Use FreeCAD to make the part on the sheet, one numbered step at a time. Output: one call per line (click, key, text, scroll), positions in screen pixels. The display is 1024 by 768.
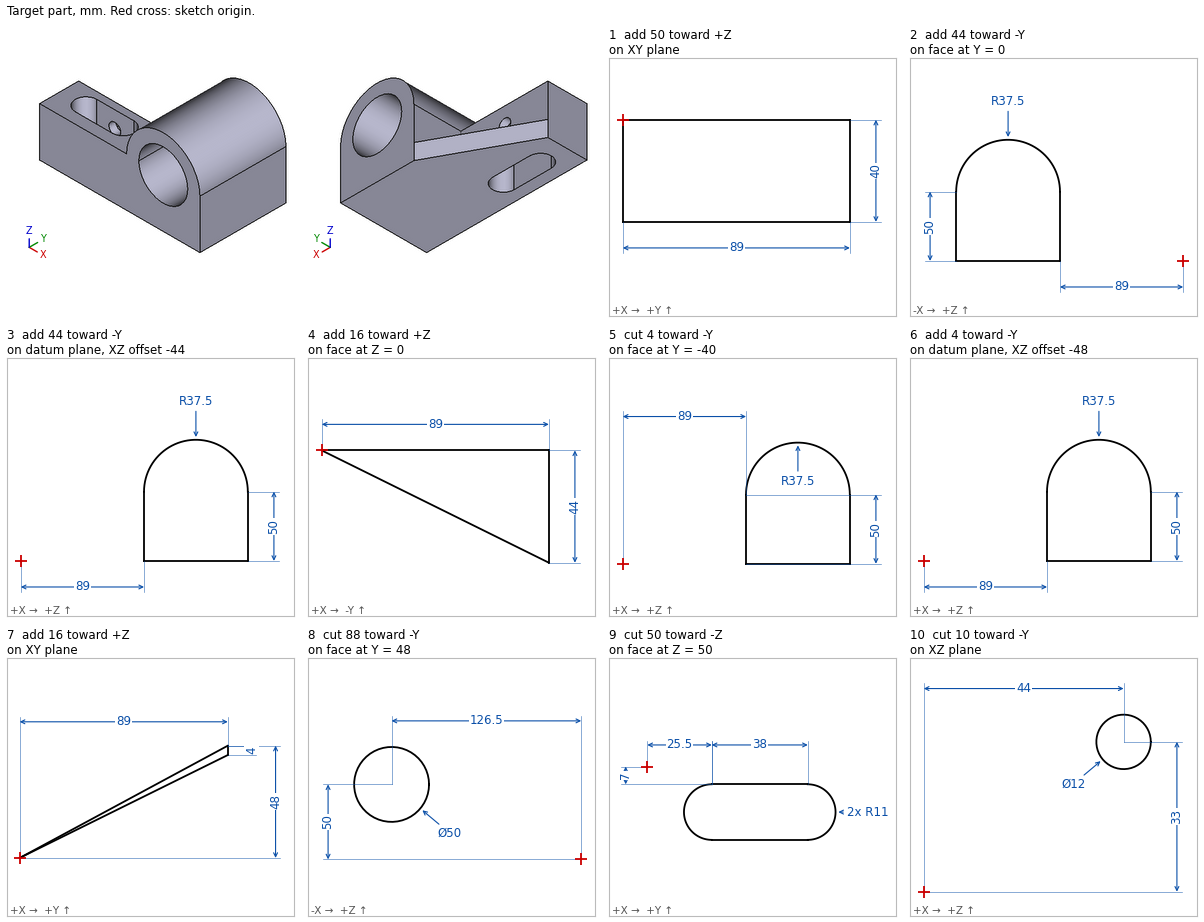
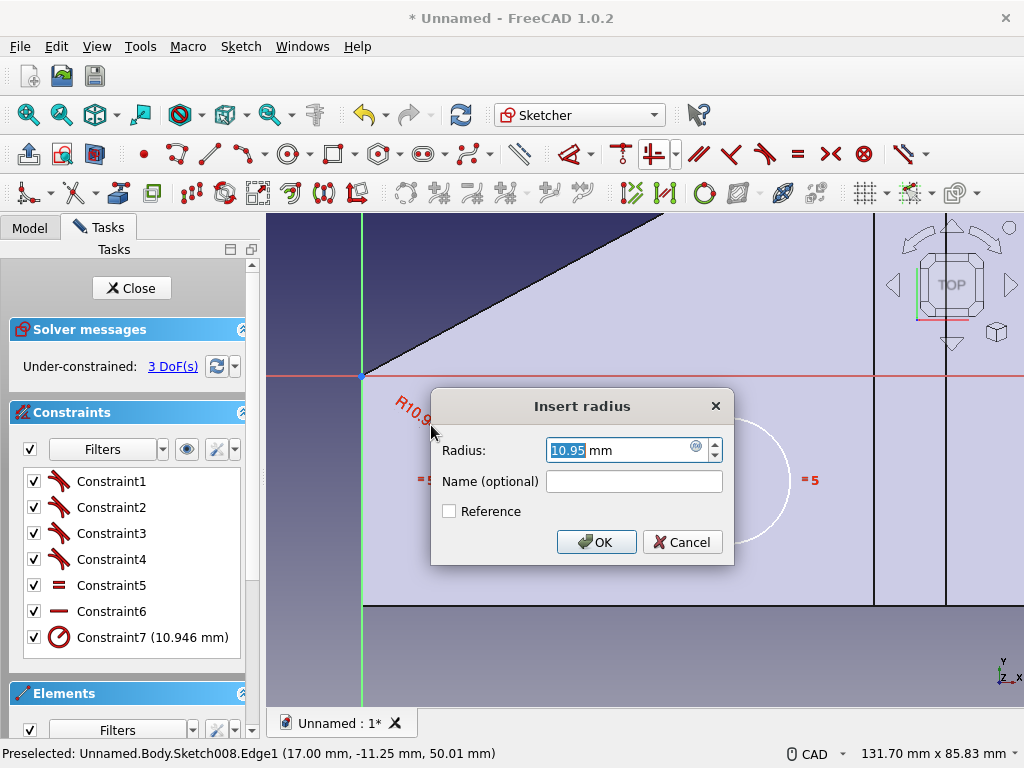
text(11)
key(Return)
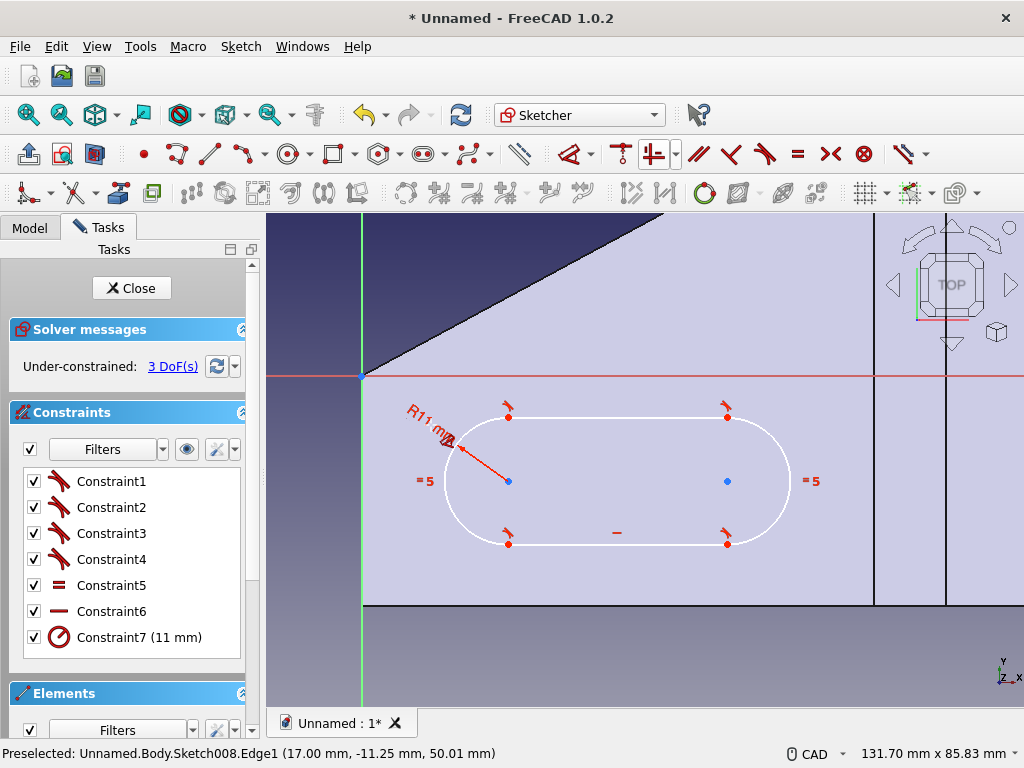
click(574, 418)
click(617, 452)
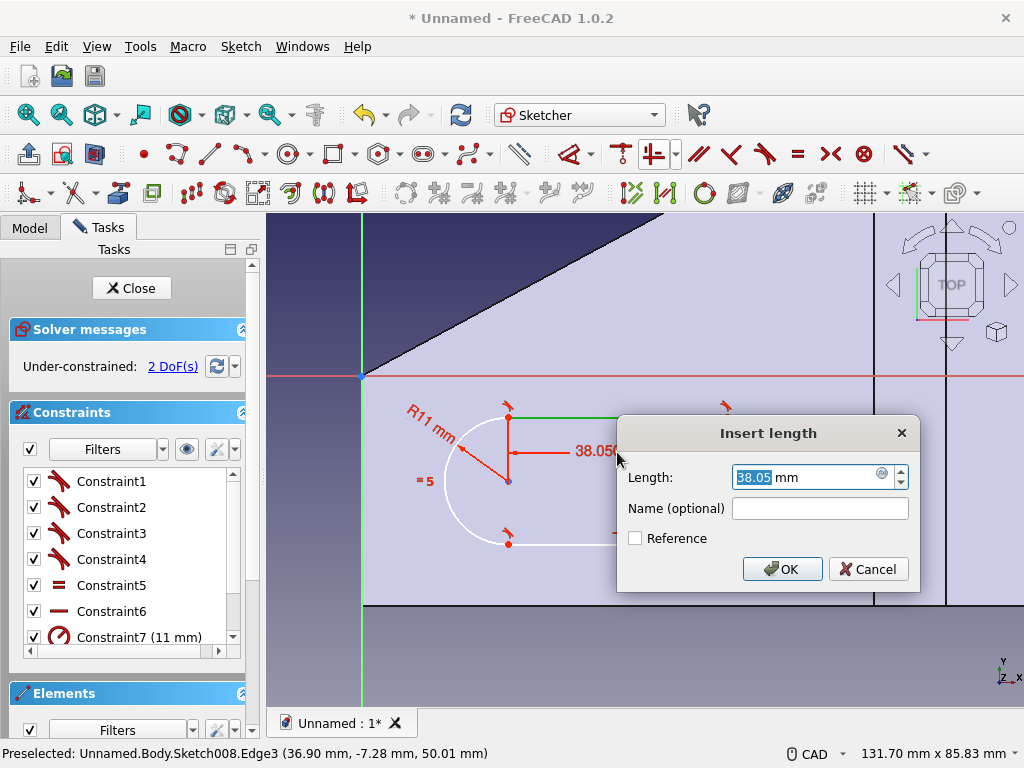
text(38)
key(Return)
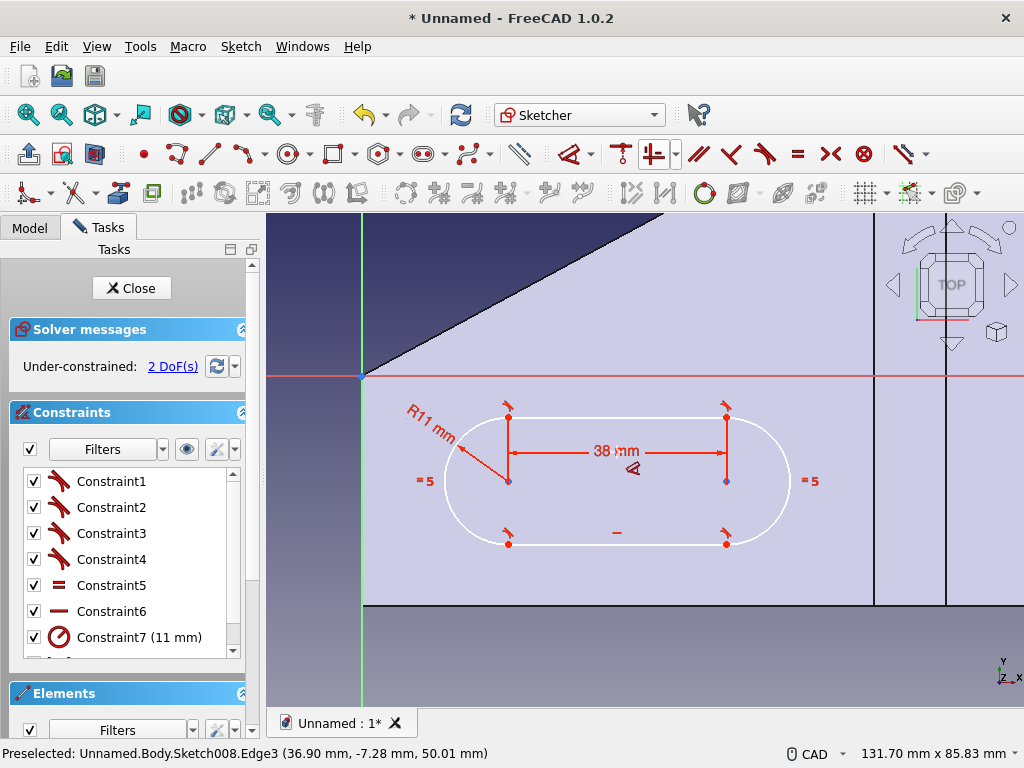
click(508, 418)
click(328, 397)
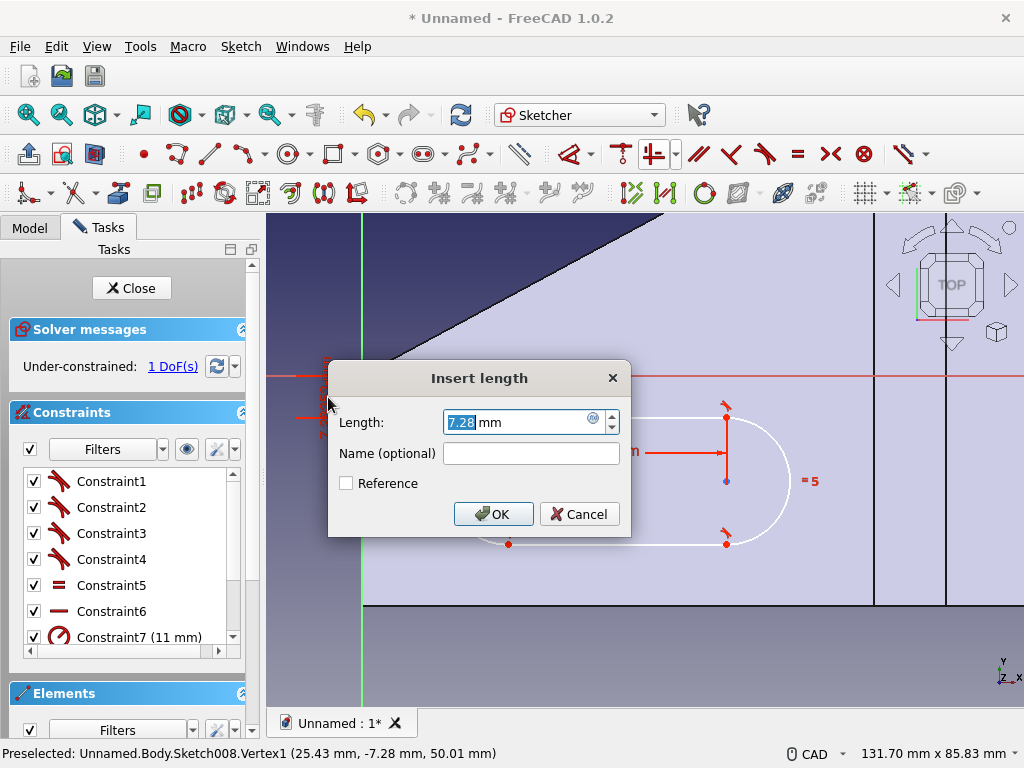
text(7)
key(Return)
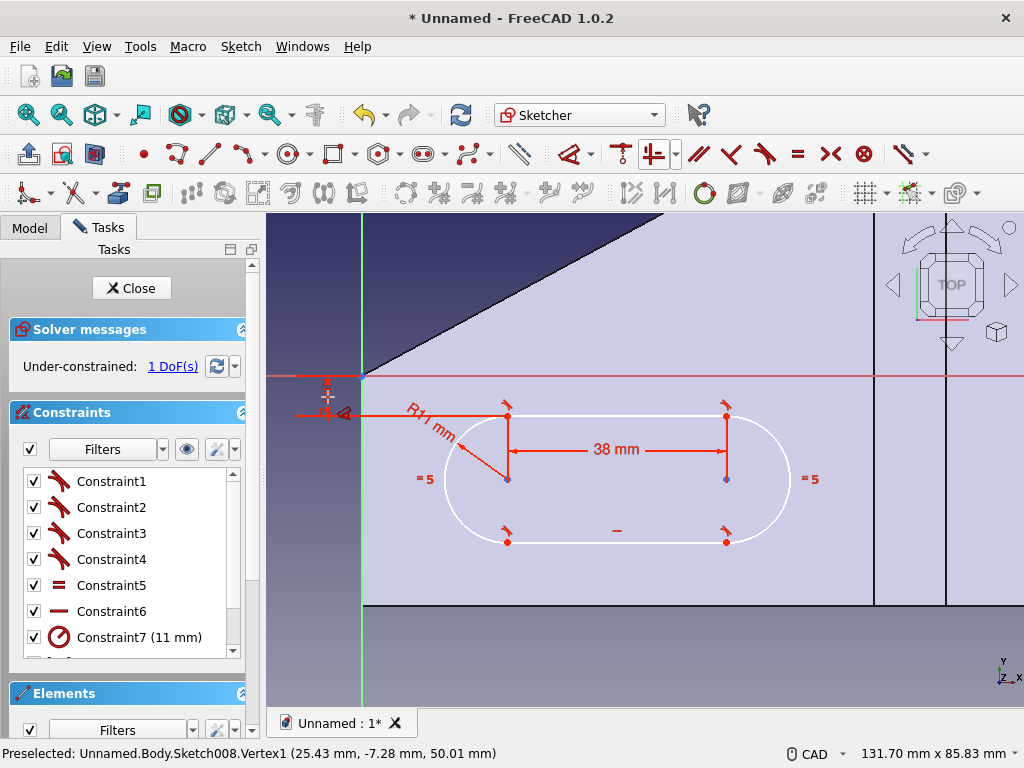
click(508, 416)
click(435, 342)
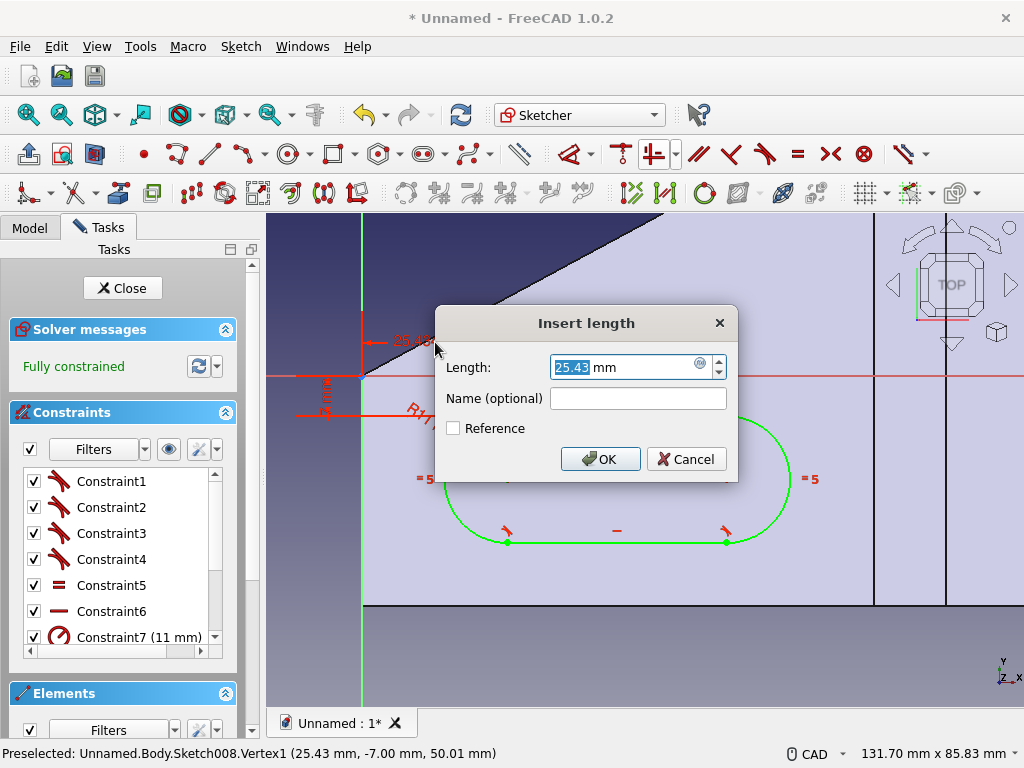
text(25.5)
key(Return)
key(Escape)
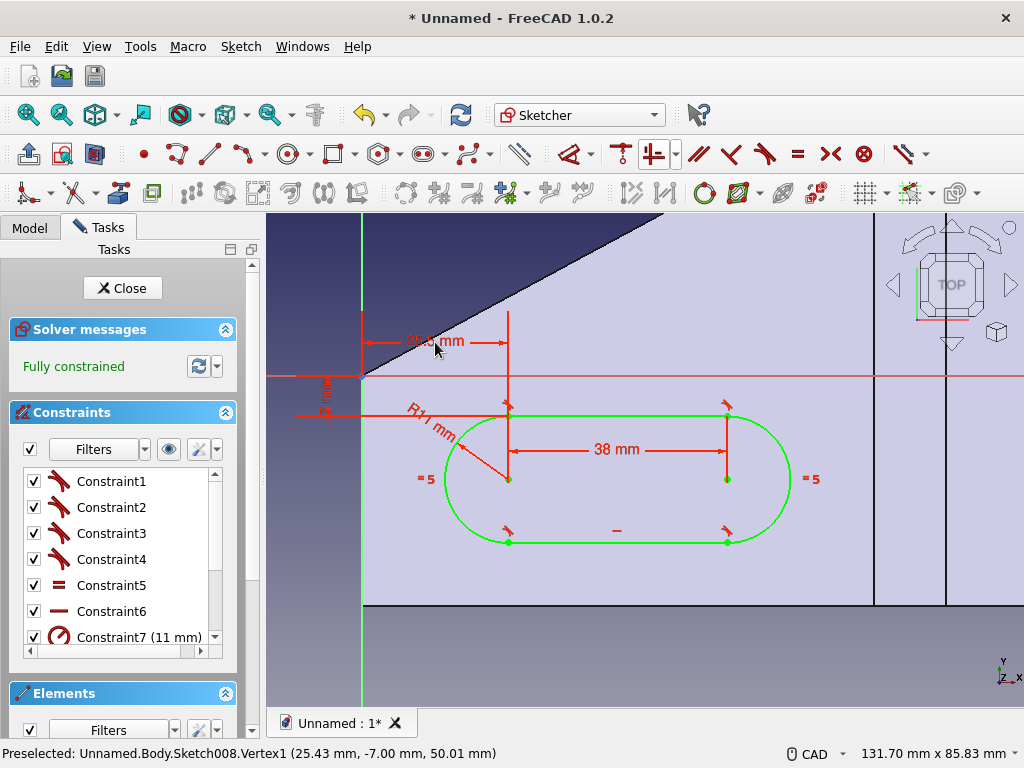
click(123, 288)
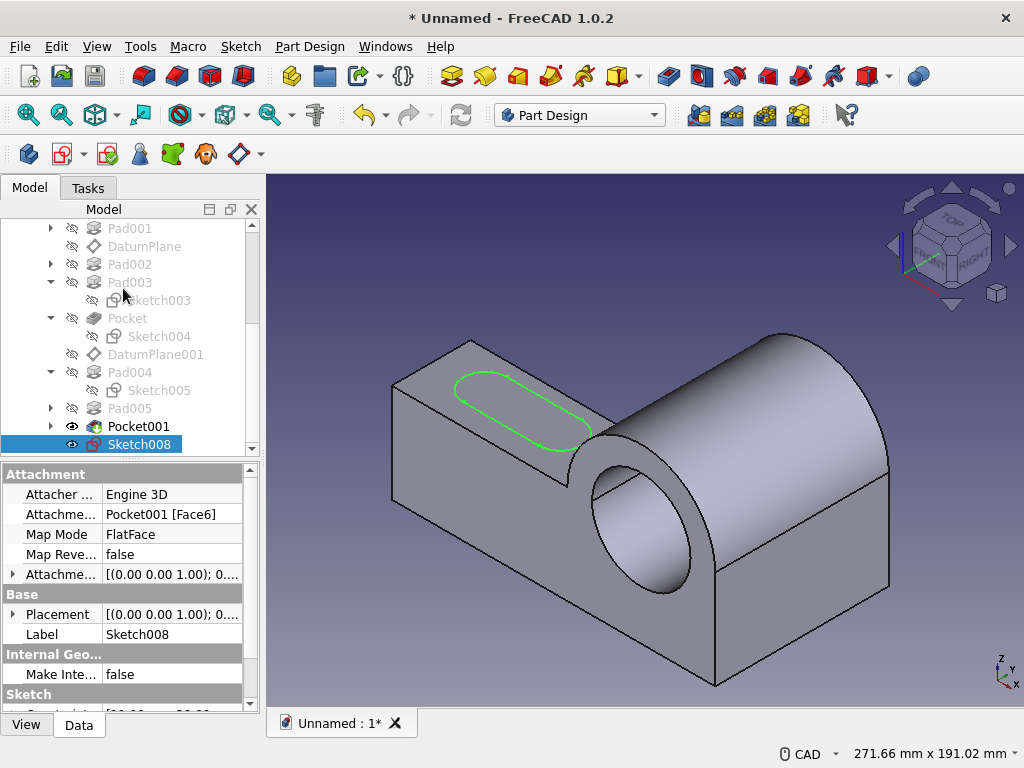
click(669, 76)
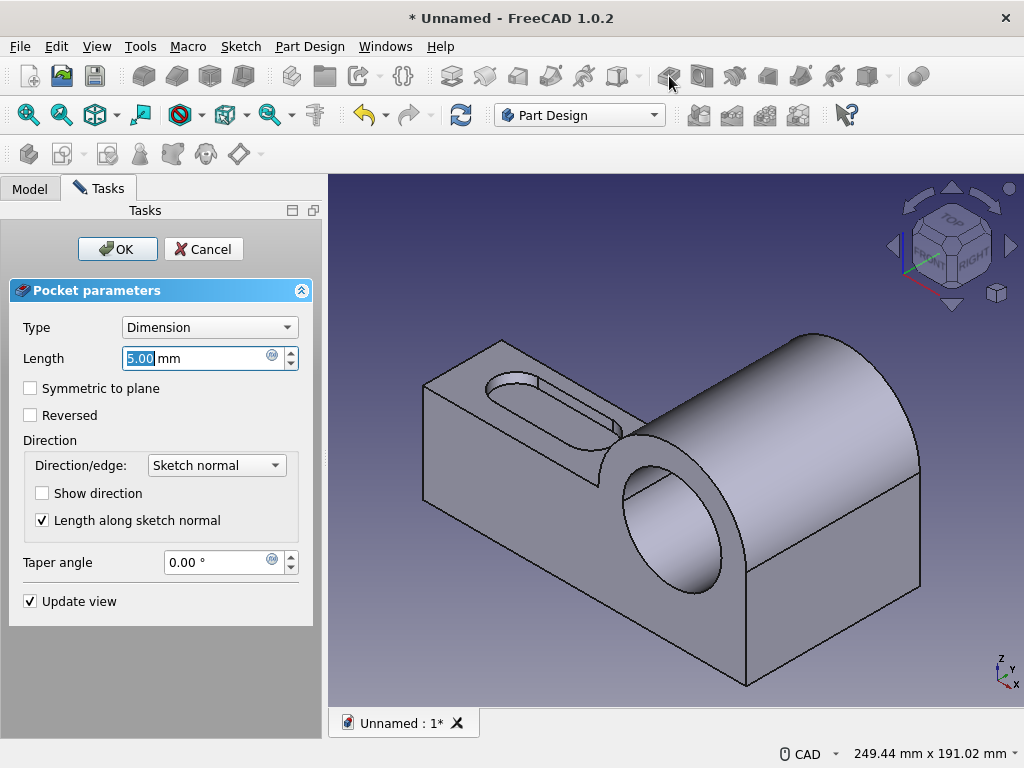
text(50)
key(Tab)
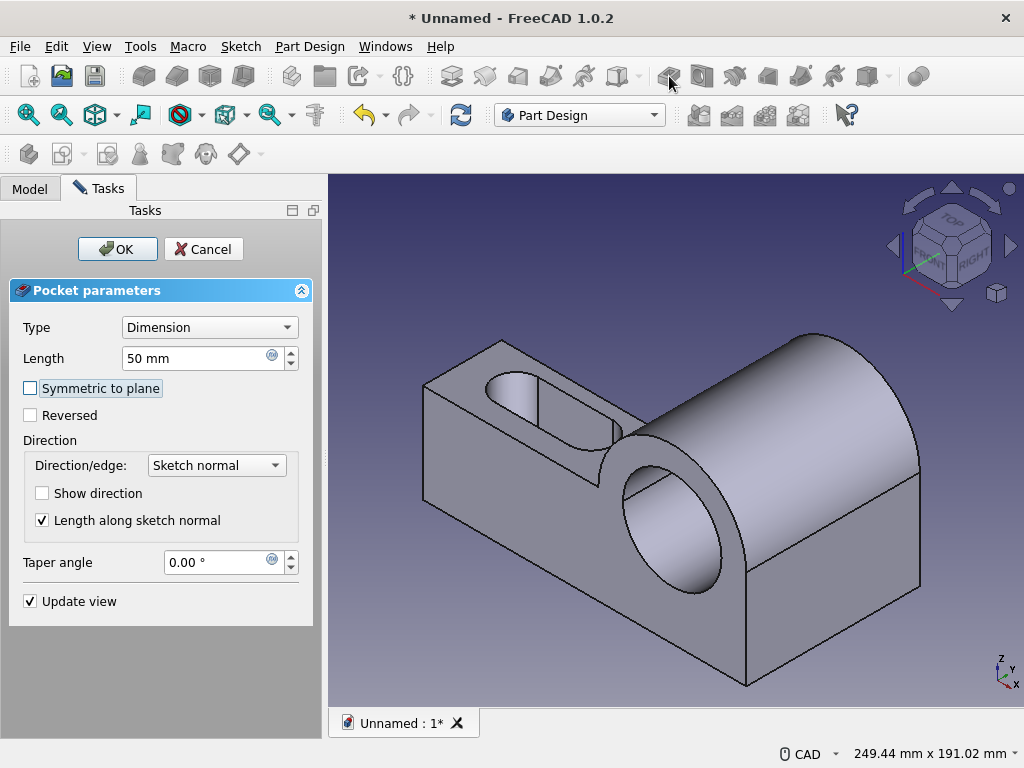
click(118, 249)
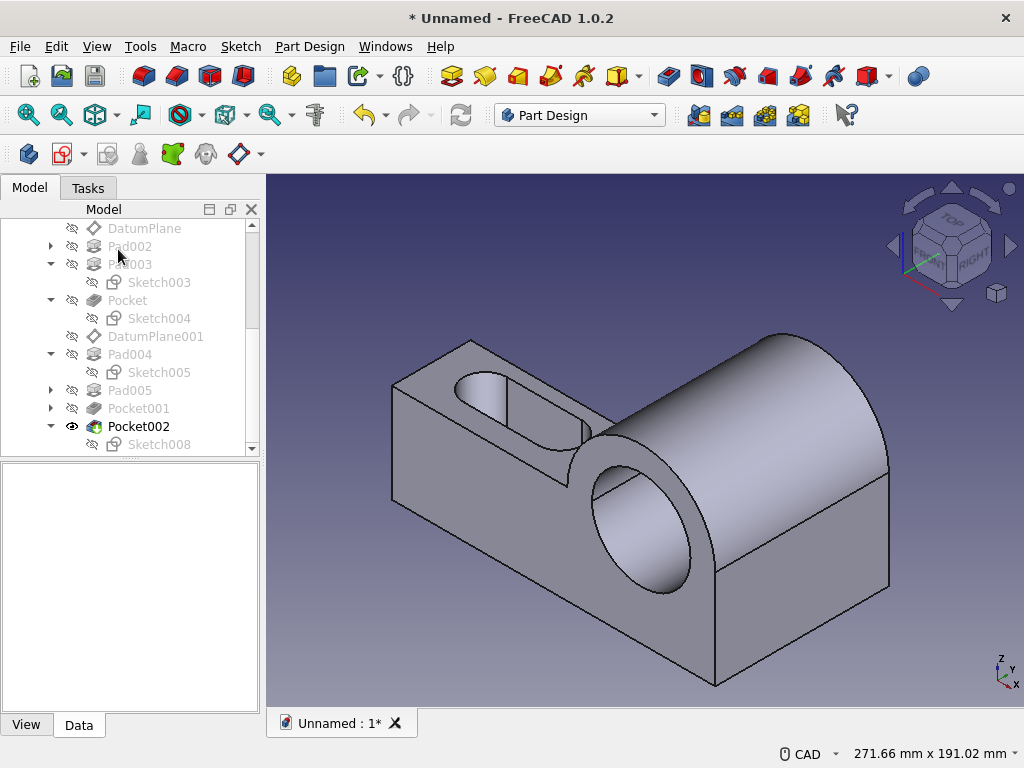
click(62, 154)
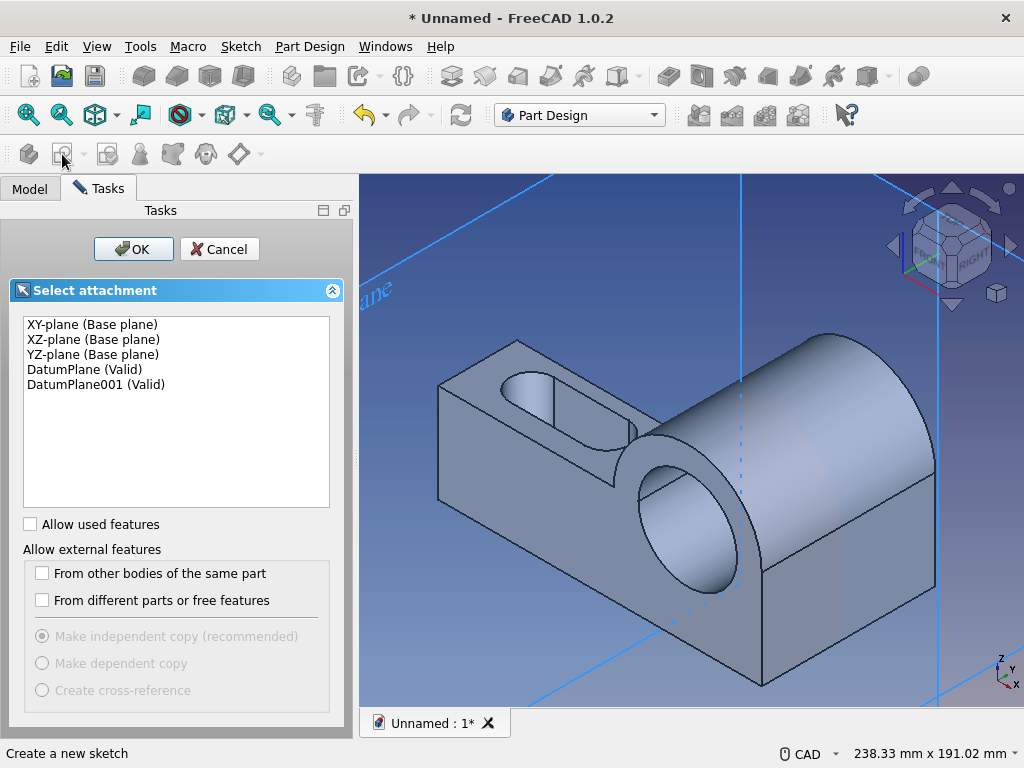
click(84, 340)